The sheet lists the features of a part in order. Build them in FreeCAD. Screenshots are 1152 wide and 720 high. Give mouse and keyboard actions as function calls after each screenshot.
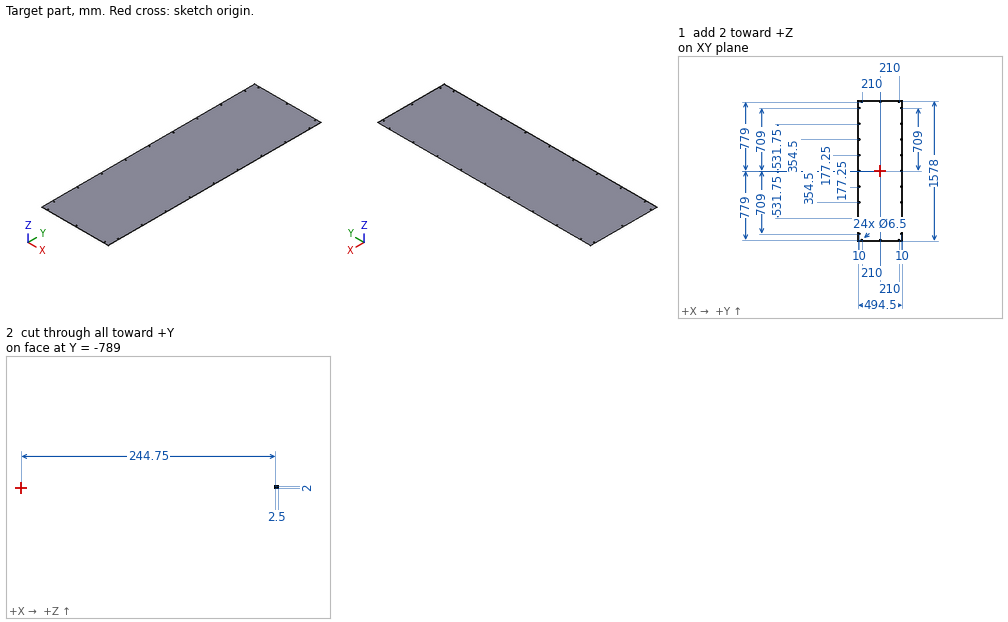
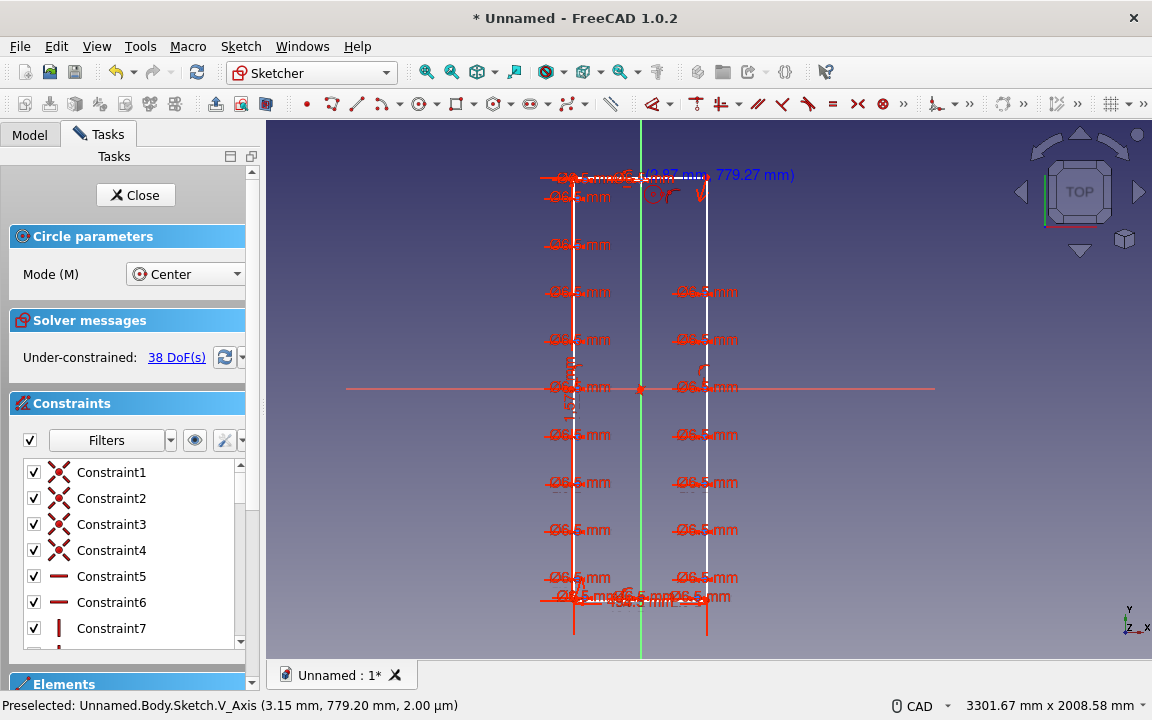
scroll(704, 247, up, 17)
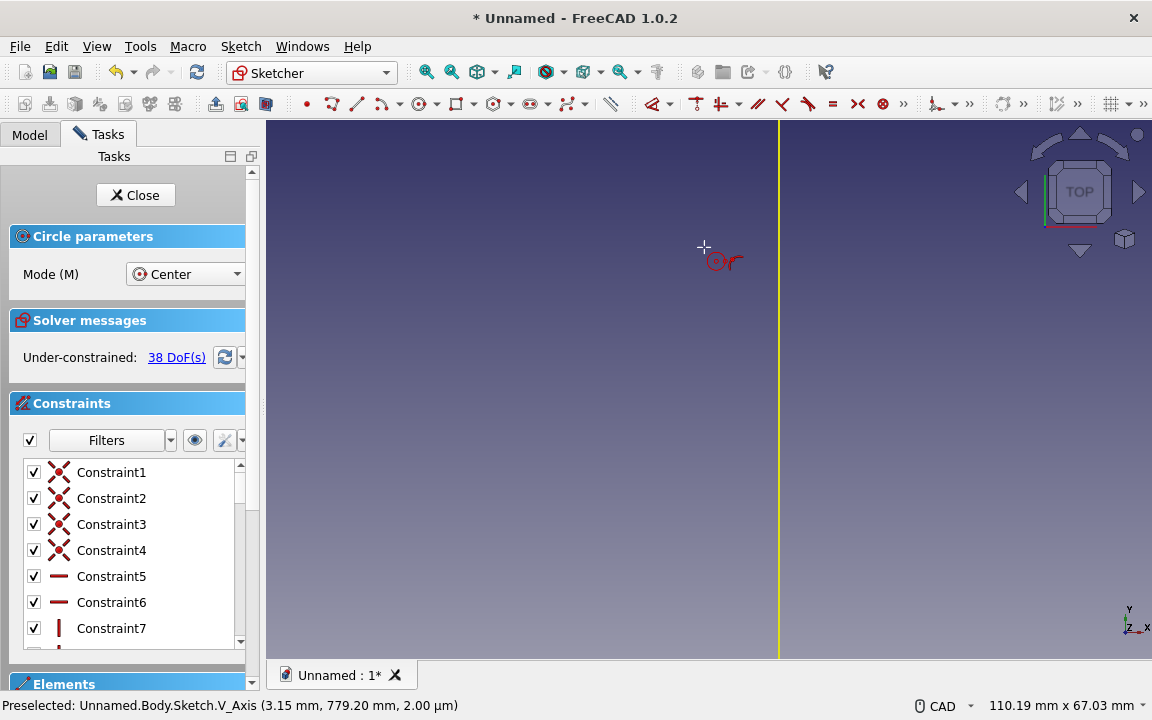
scroll(704, 247, down, 17)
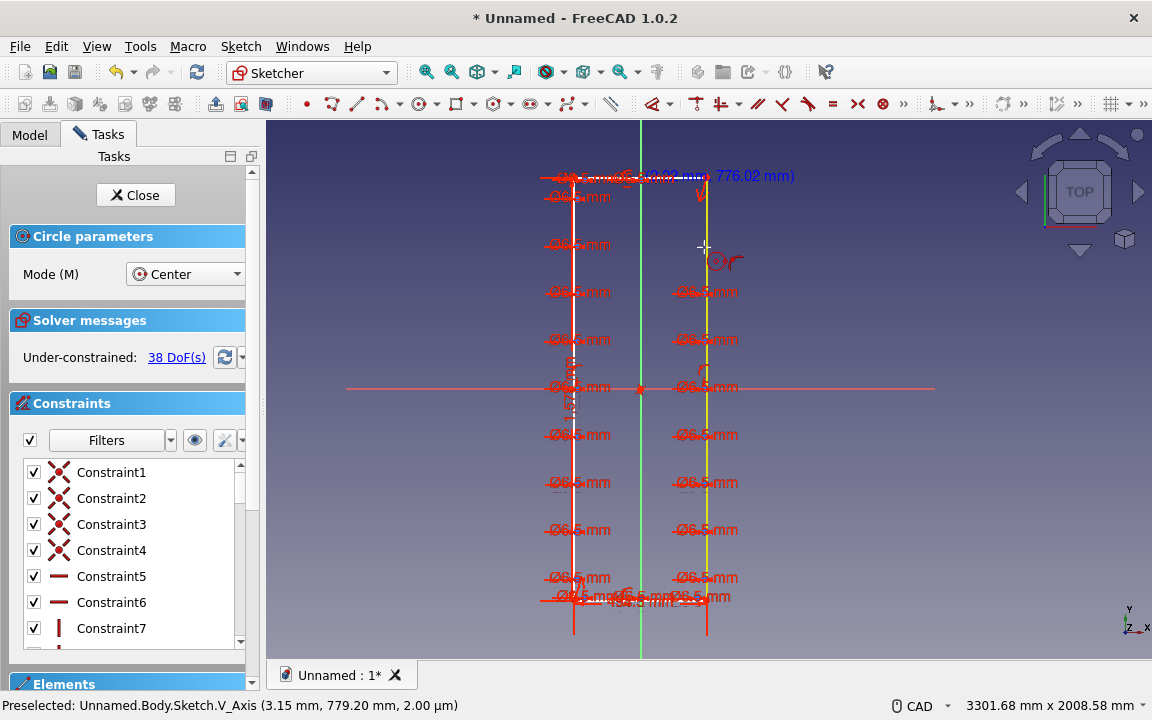
scroll(704, 247, up, 9)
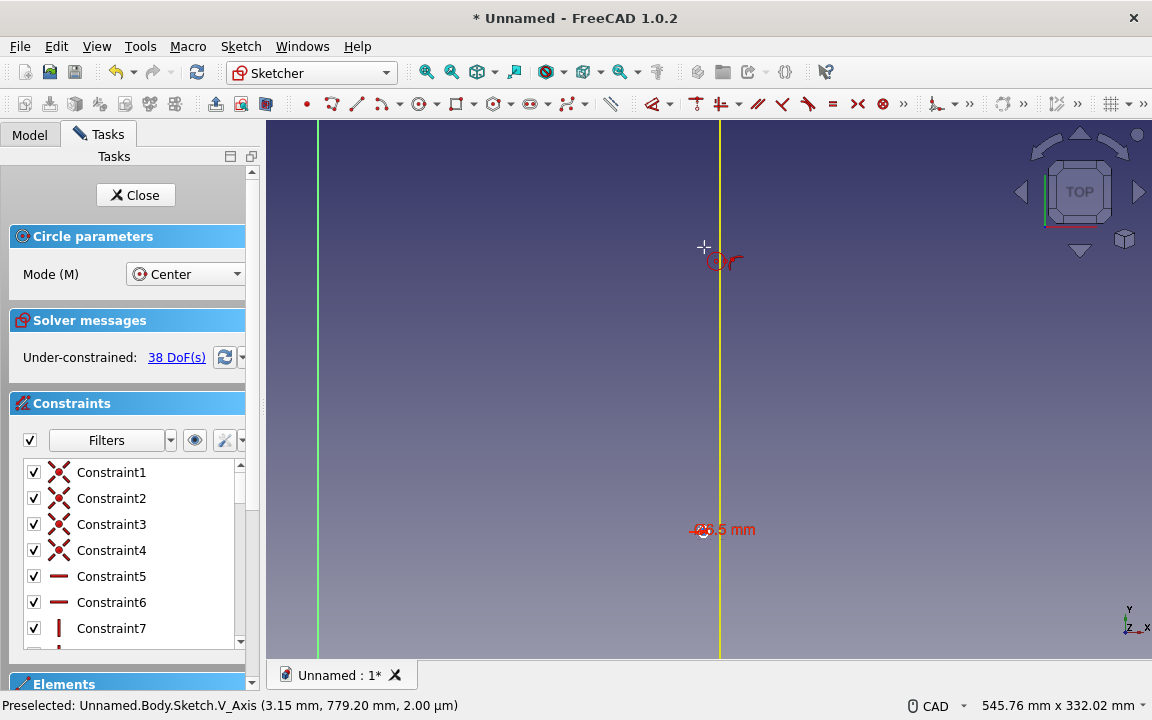
click(703, 243)
move(700, 240)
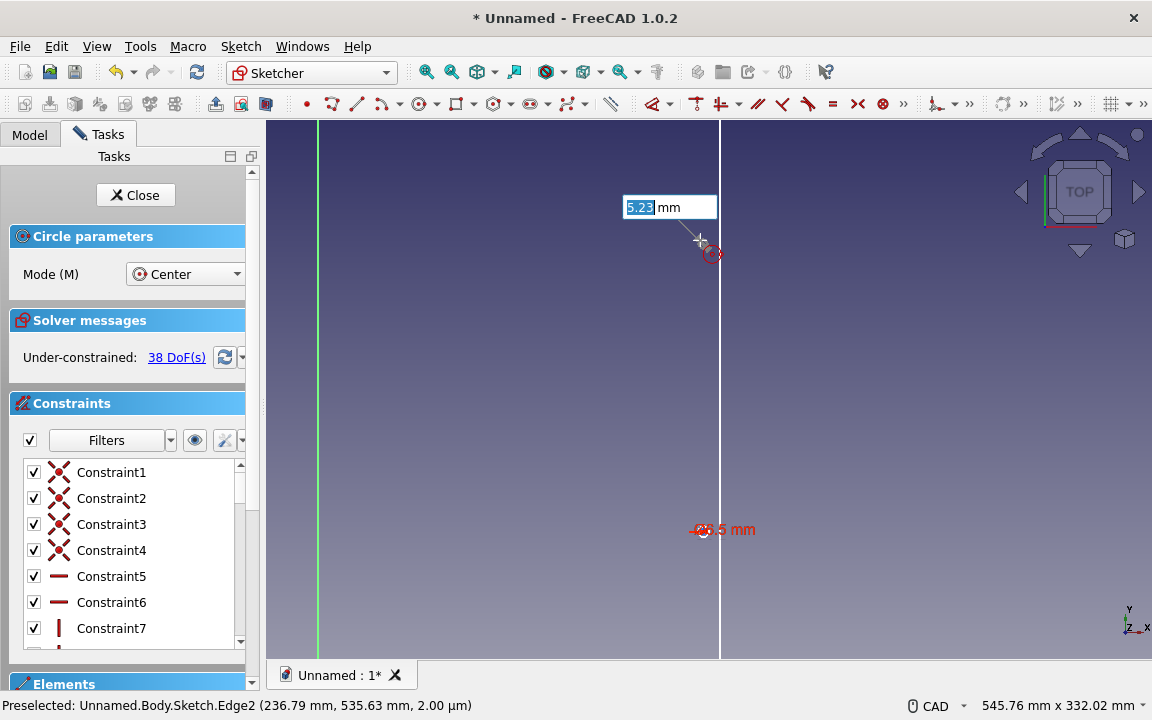
text(6.5)
key(Return)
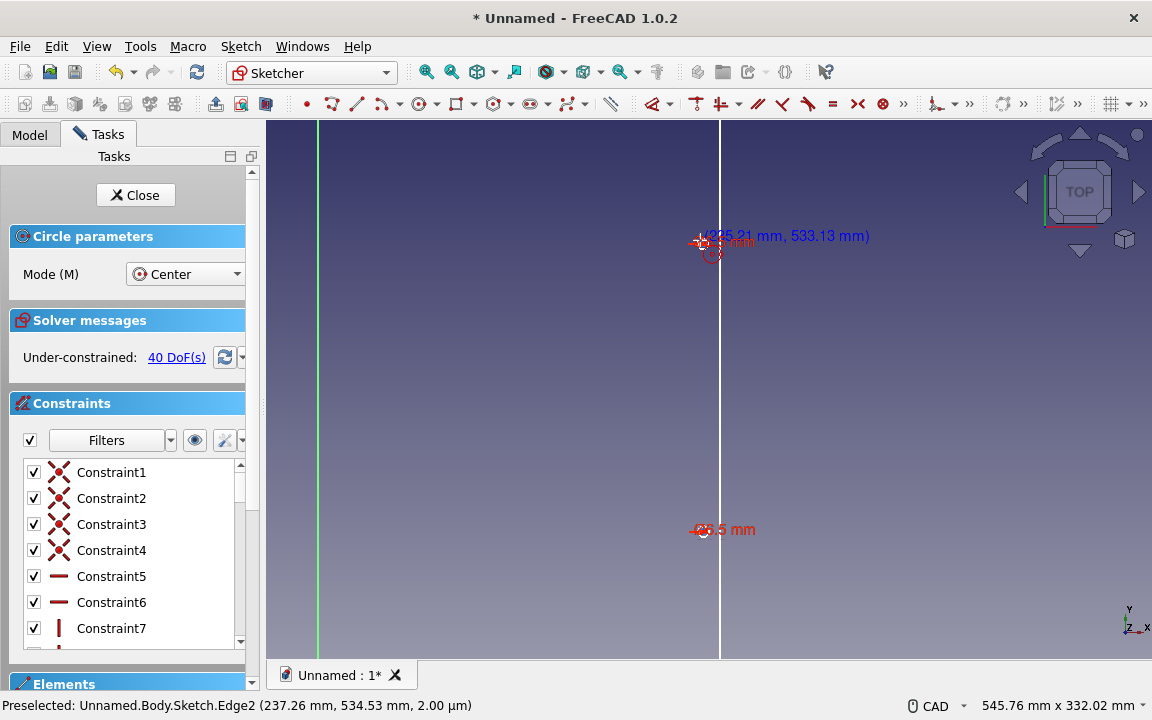
scroll(691, 277, down, 10)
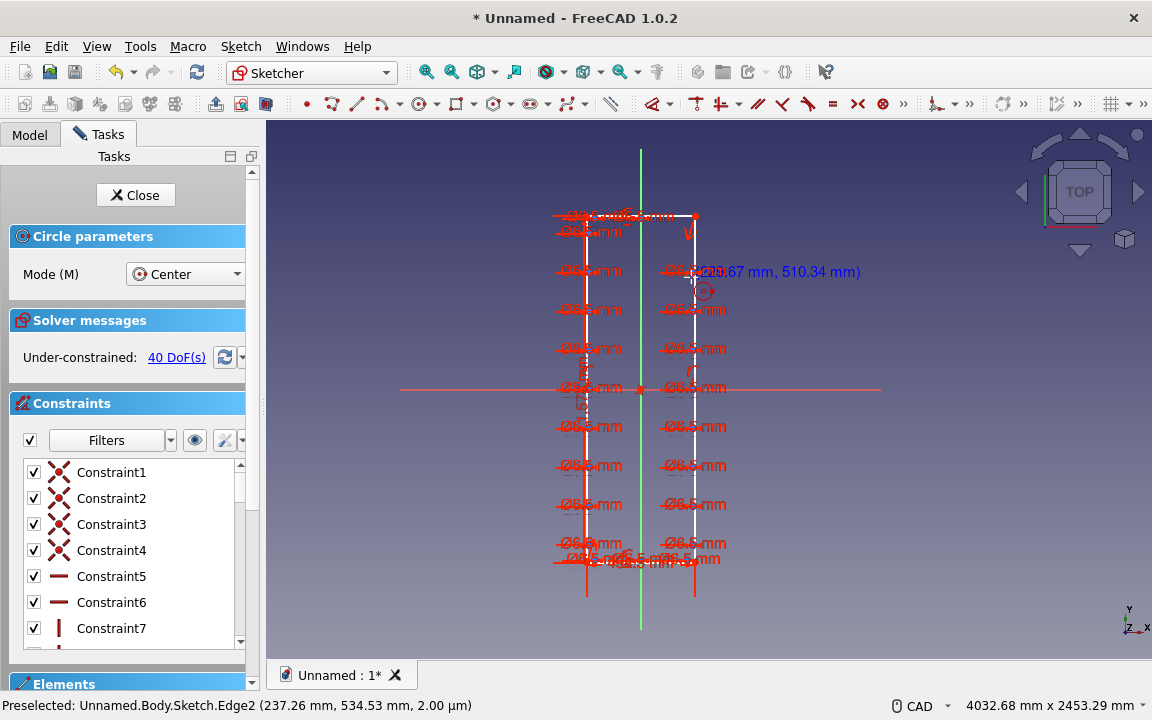
scroll(687, 218, up, 18)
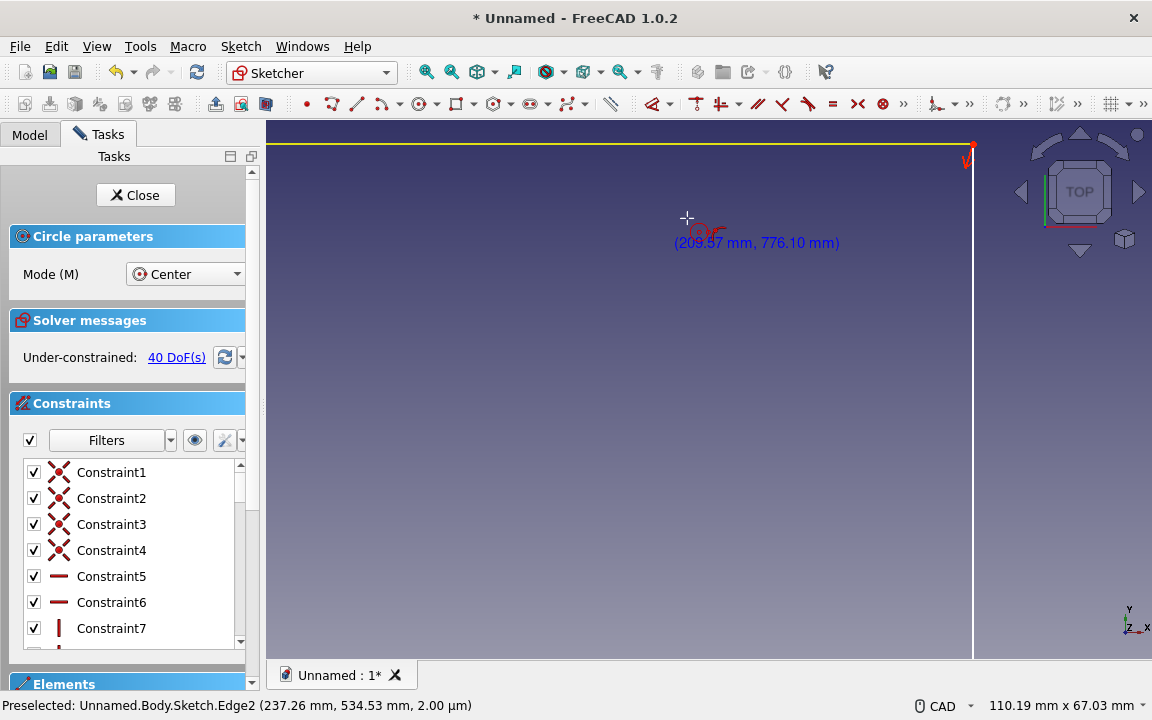
scroll(698, 179, down, 17)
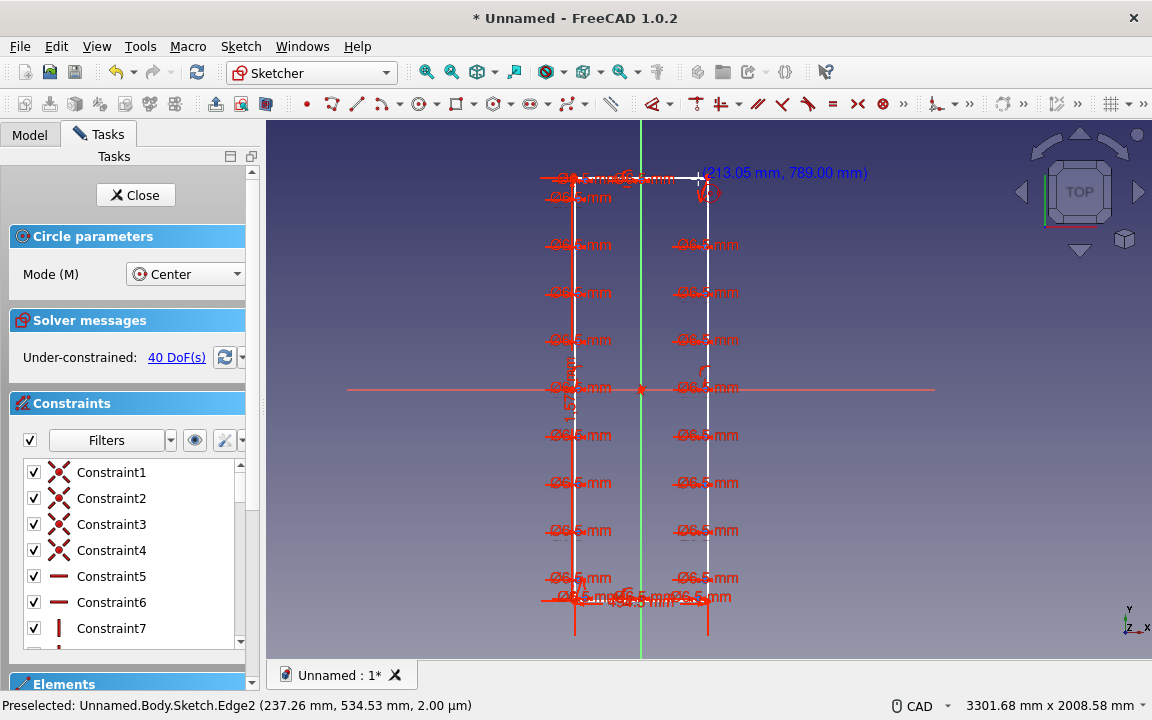
scroll(698, 181, up, 9)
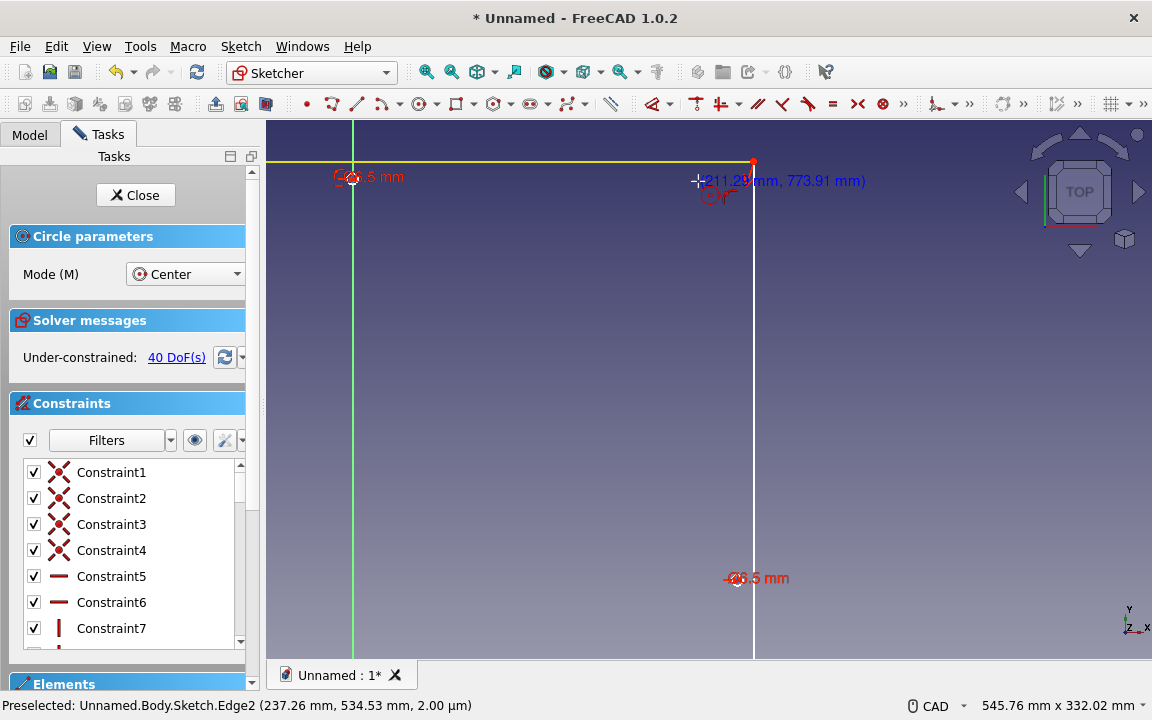
click(693, 178)
move(697, 182)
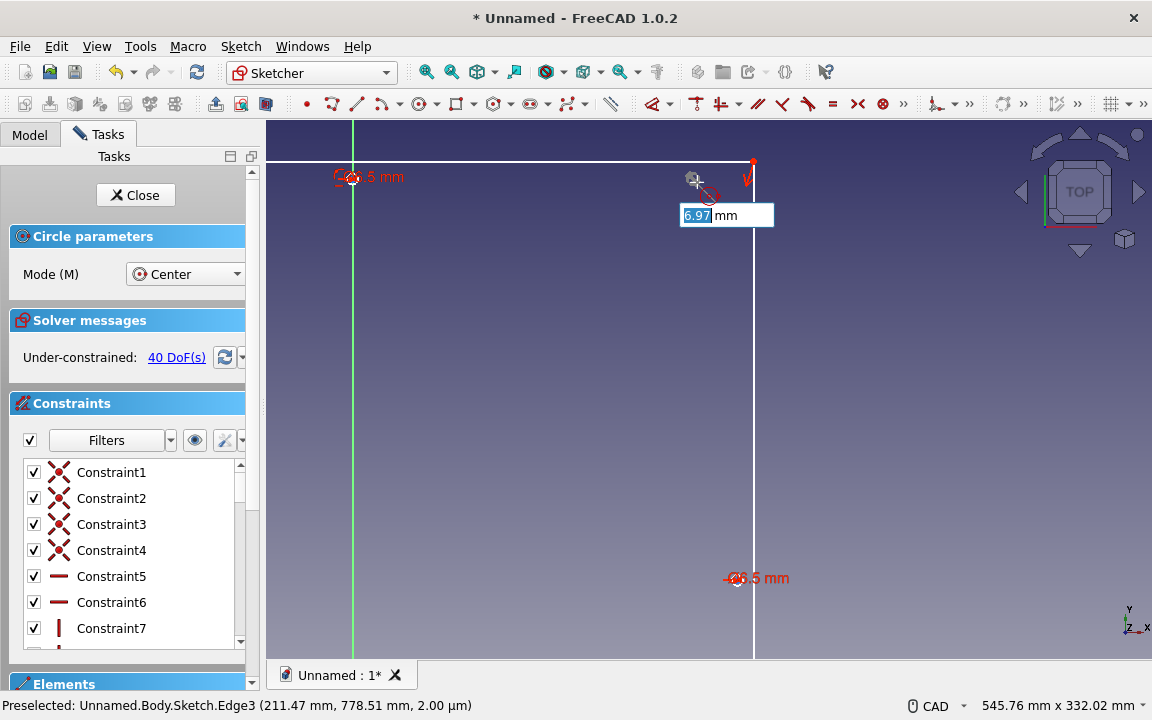
text(6.5)
key(Return)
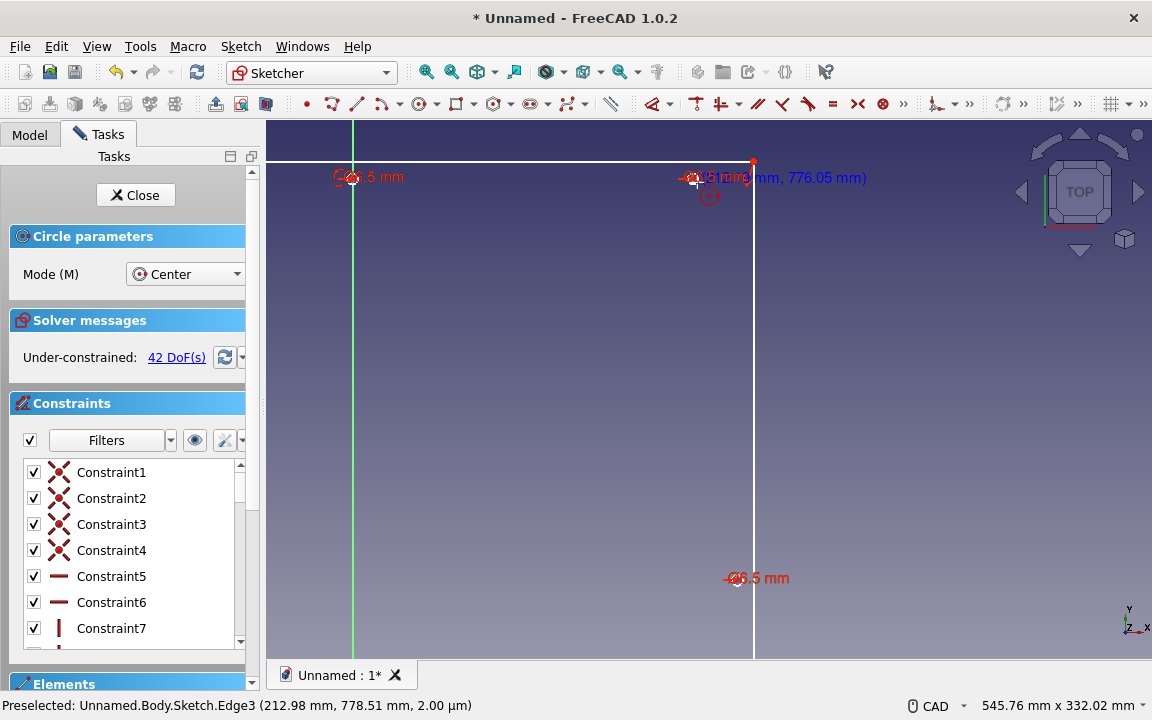
scroll(738, 292, up, 8)